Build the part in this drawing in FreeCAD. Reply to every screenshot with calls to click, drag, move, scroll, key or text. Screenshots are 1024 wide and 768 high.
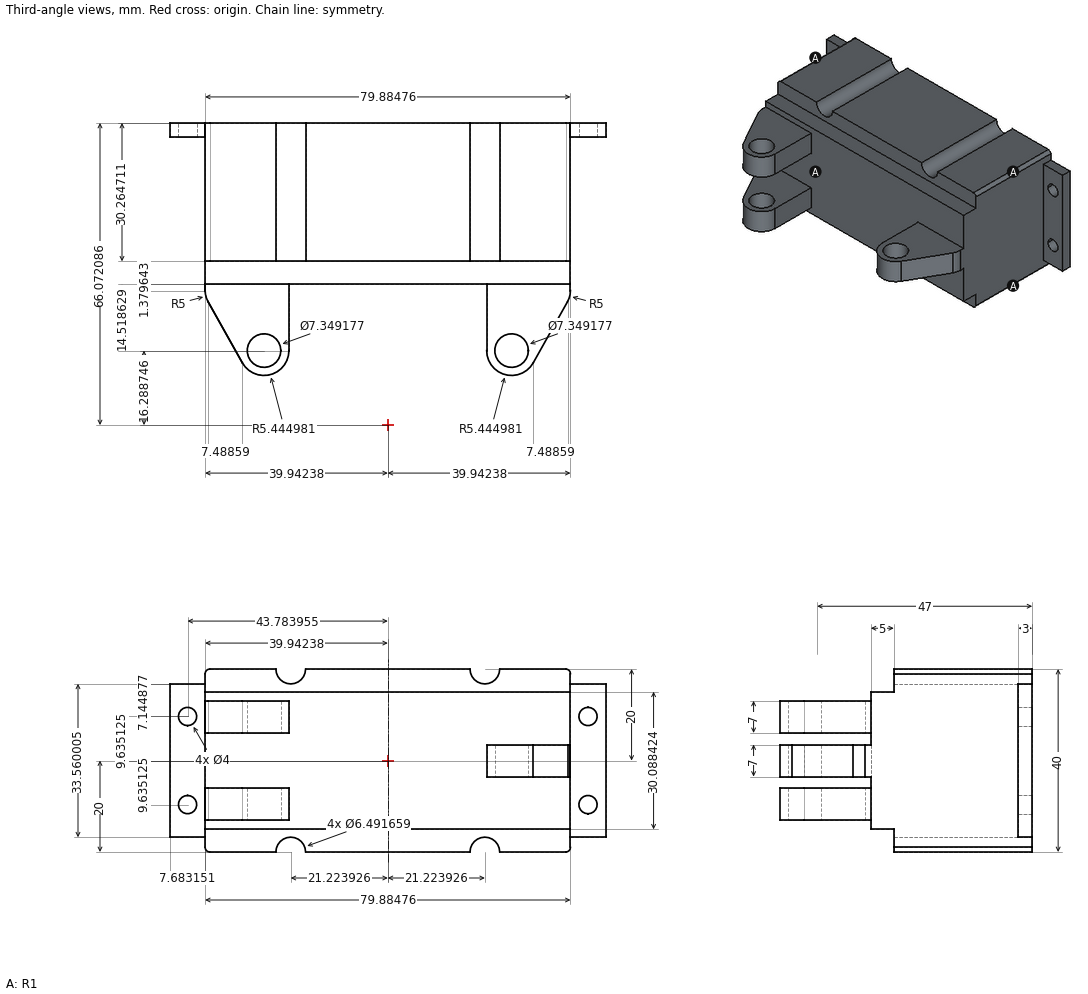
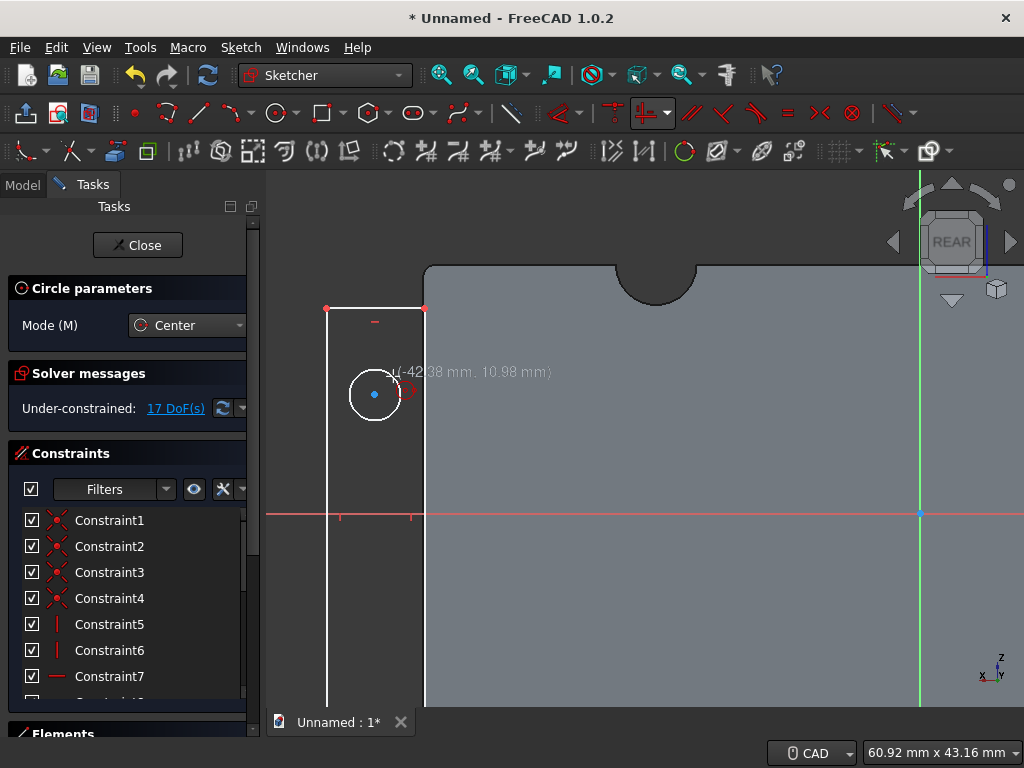
click(375, 633)
click(393, 616)
key(Escape)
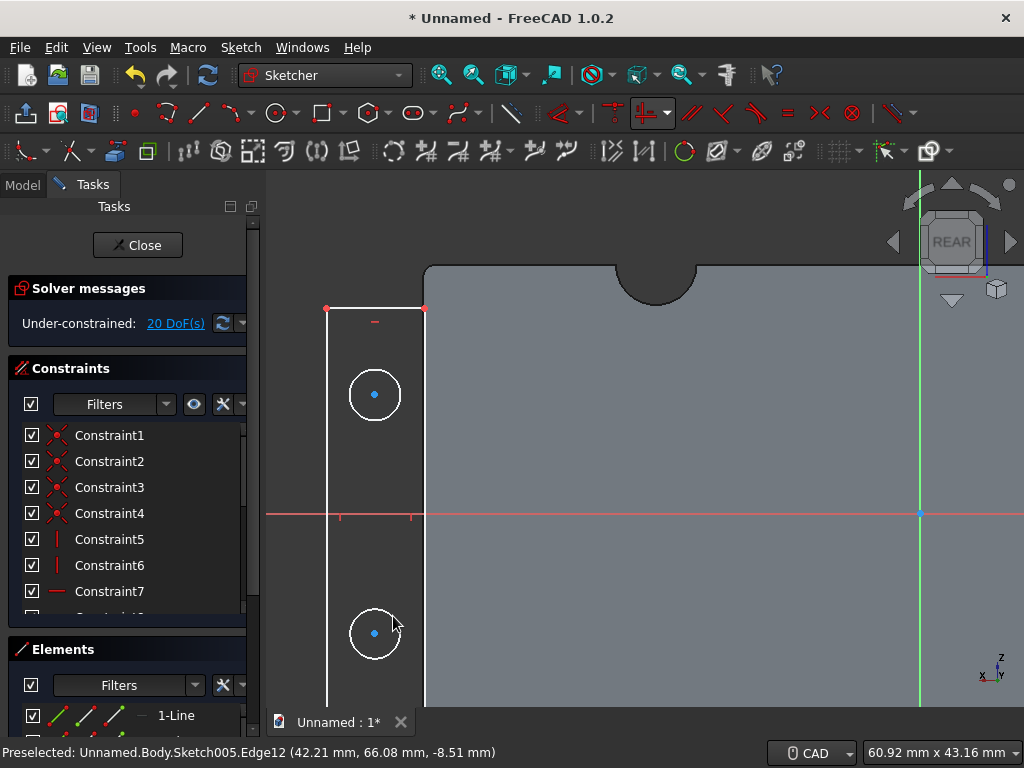
scroll(376, 395, down, 5)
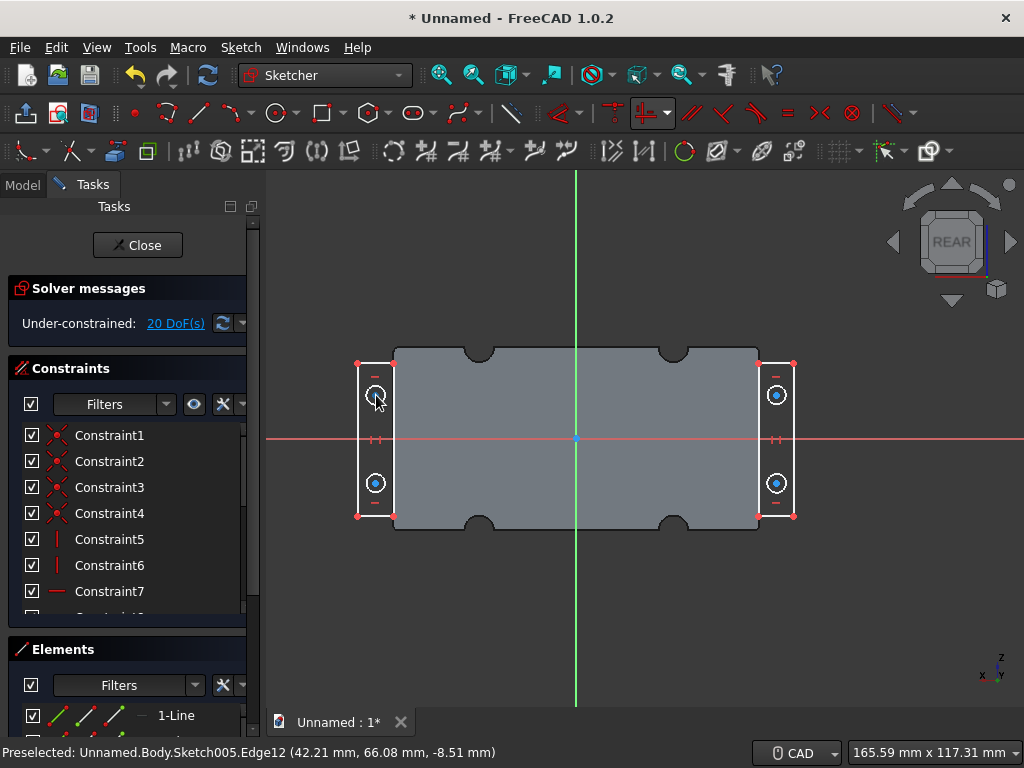
scroll(783, 389, up, 3)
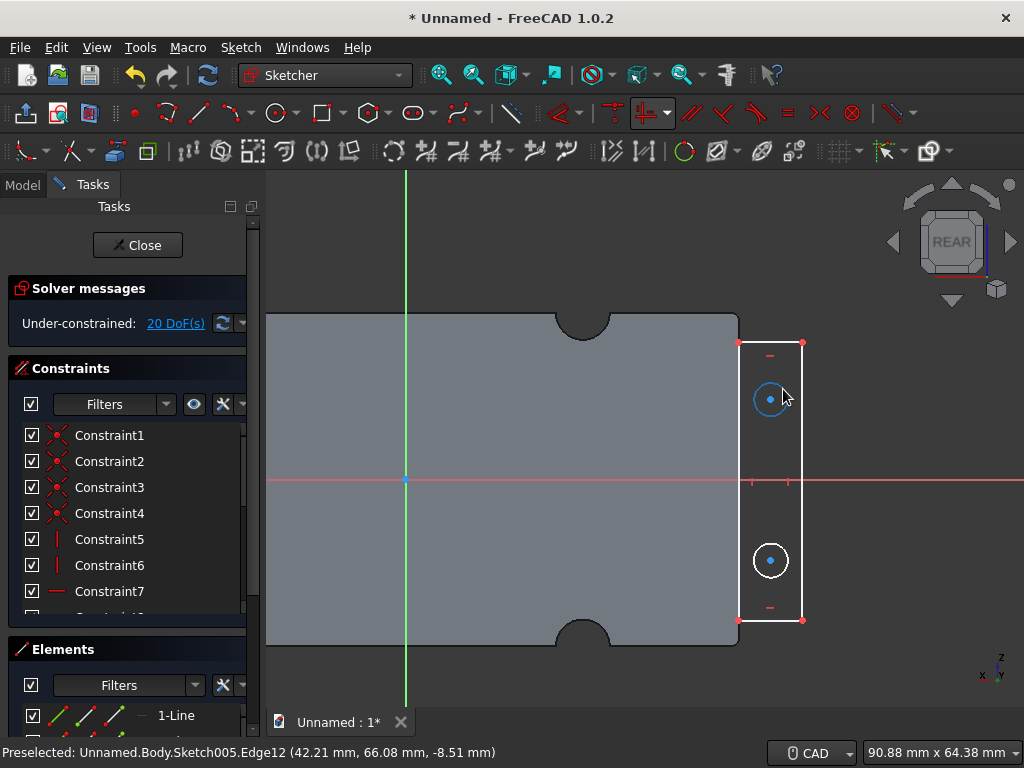
click(783, 388)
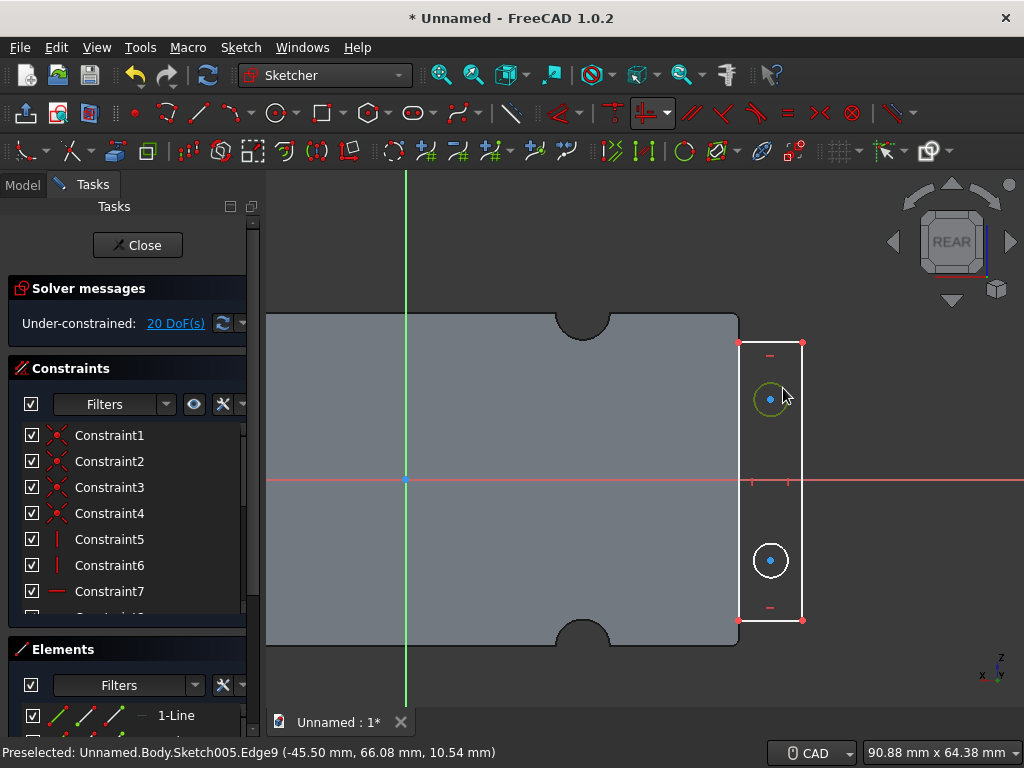
click(783, 548)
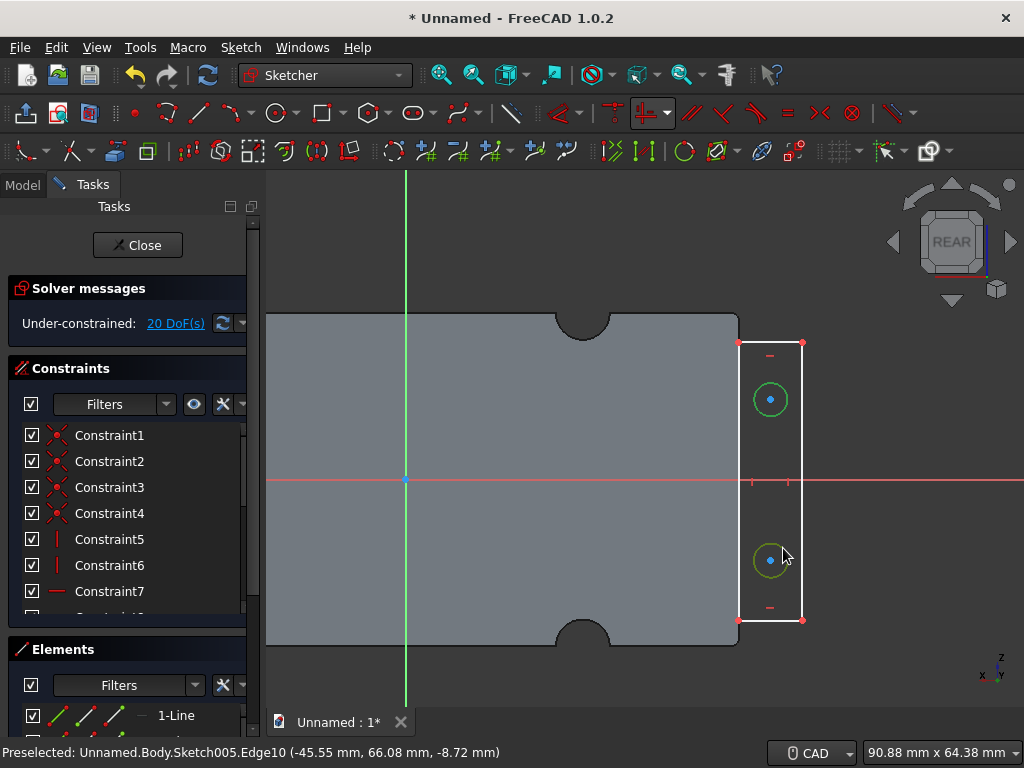
scroll(784, 389, down, 3)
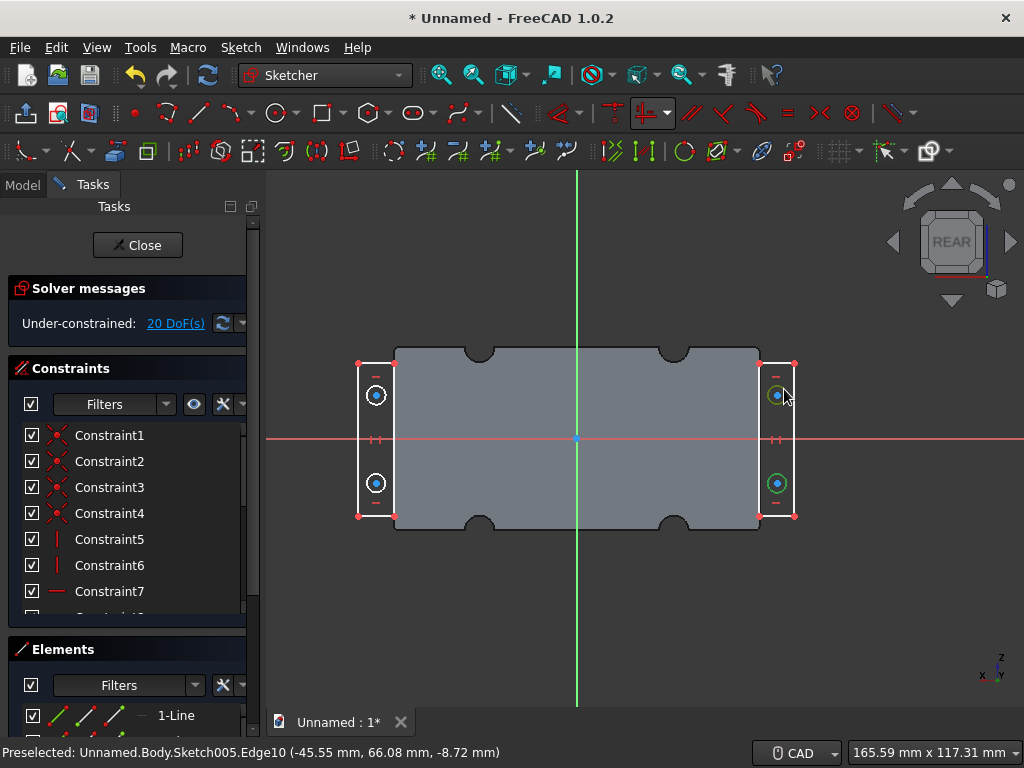
scroll(383, 389, up, 2)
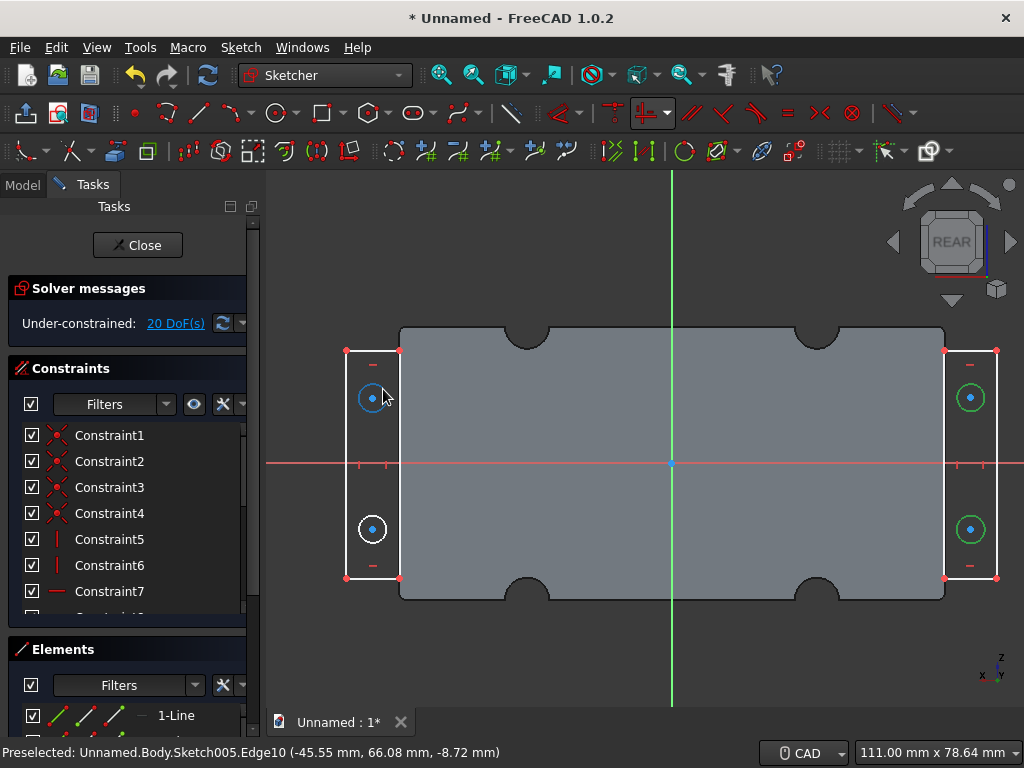
click(383, 388)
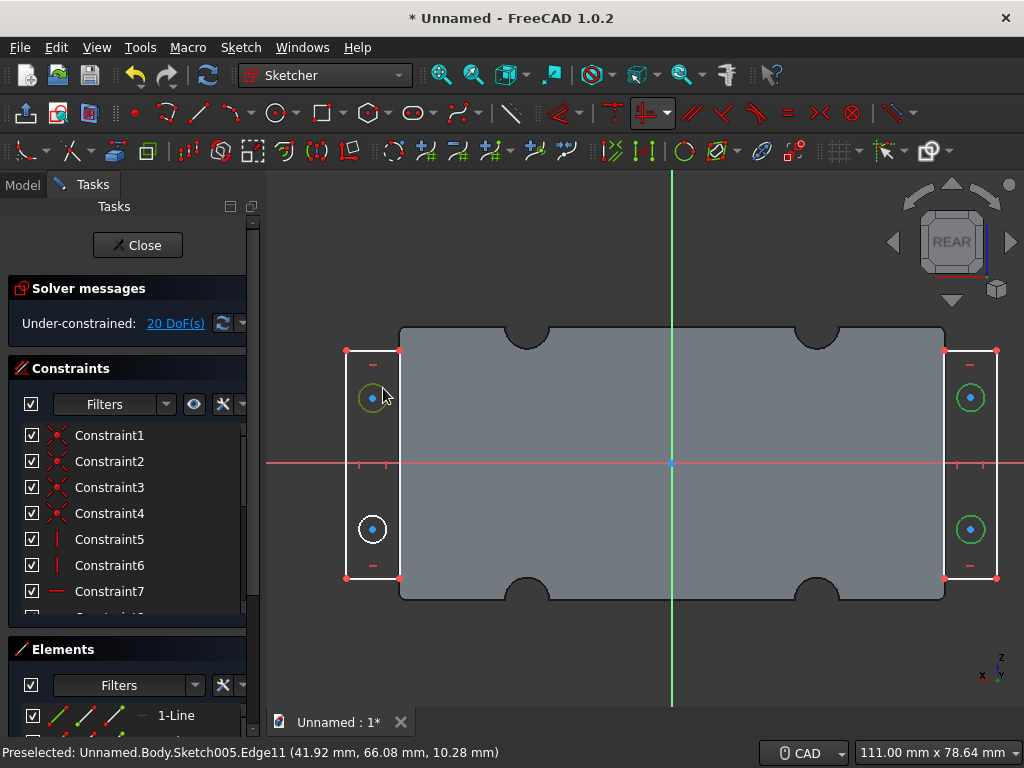
click(382, 520)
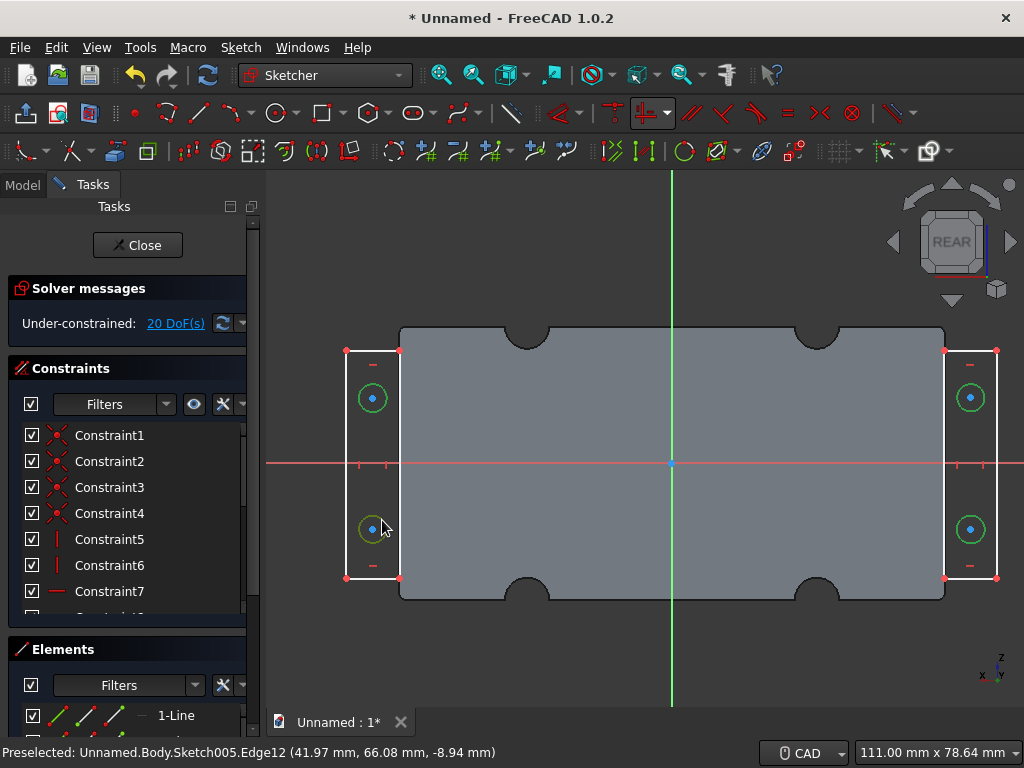
click(788, 114)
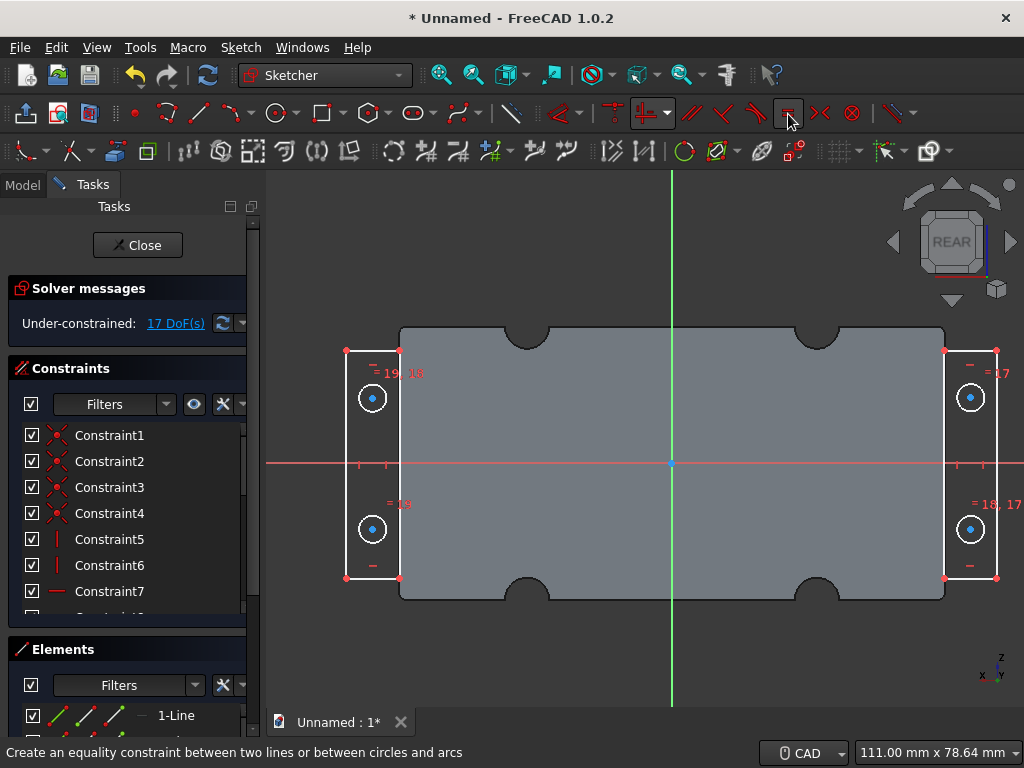
scroll(382, 388, down, 2)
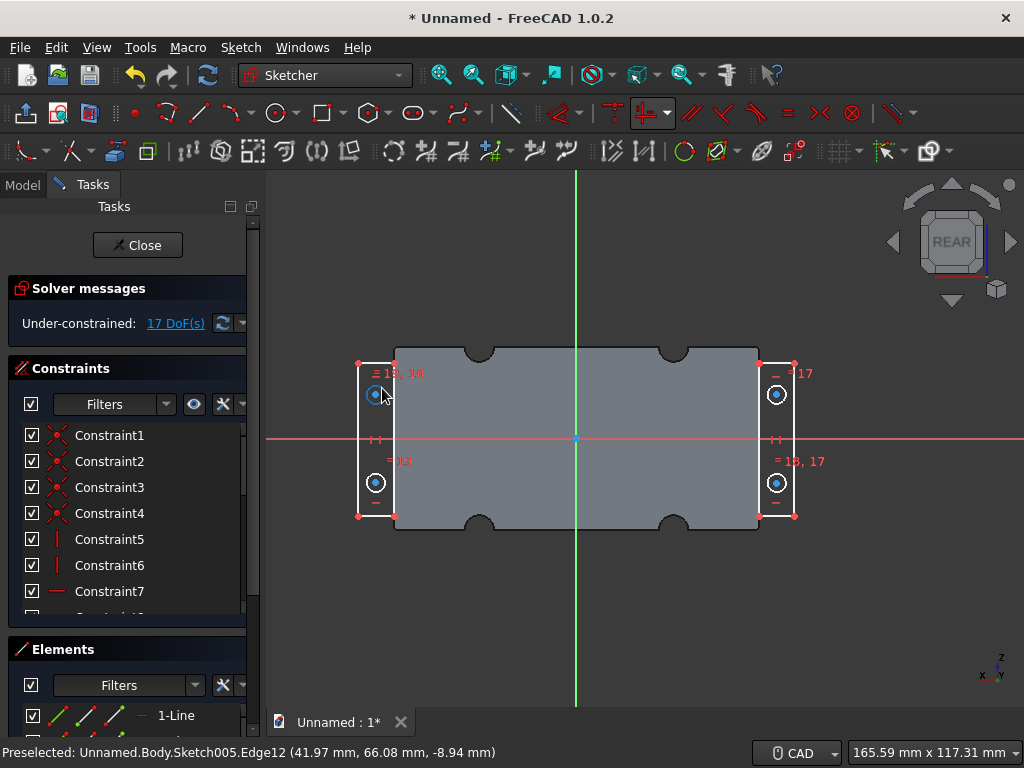
click(777, 395)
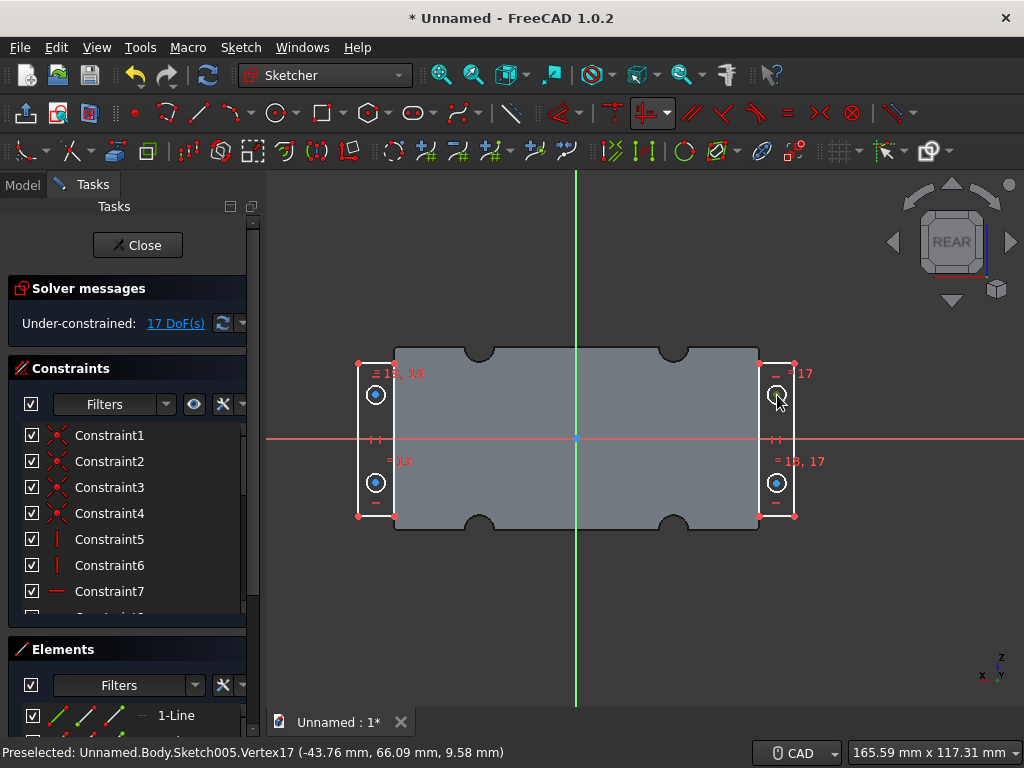
click(777, 483)